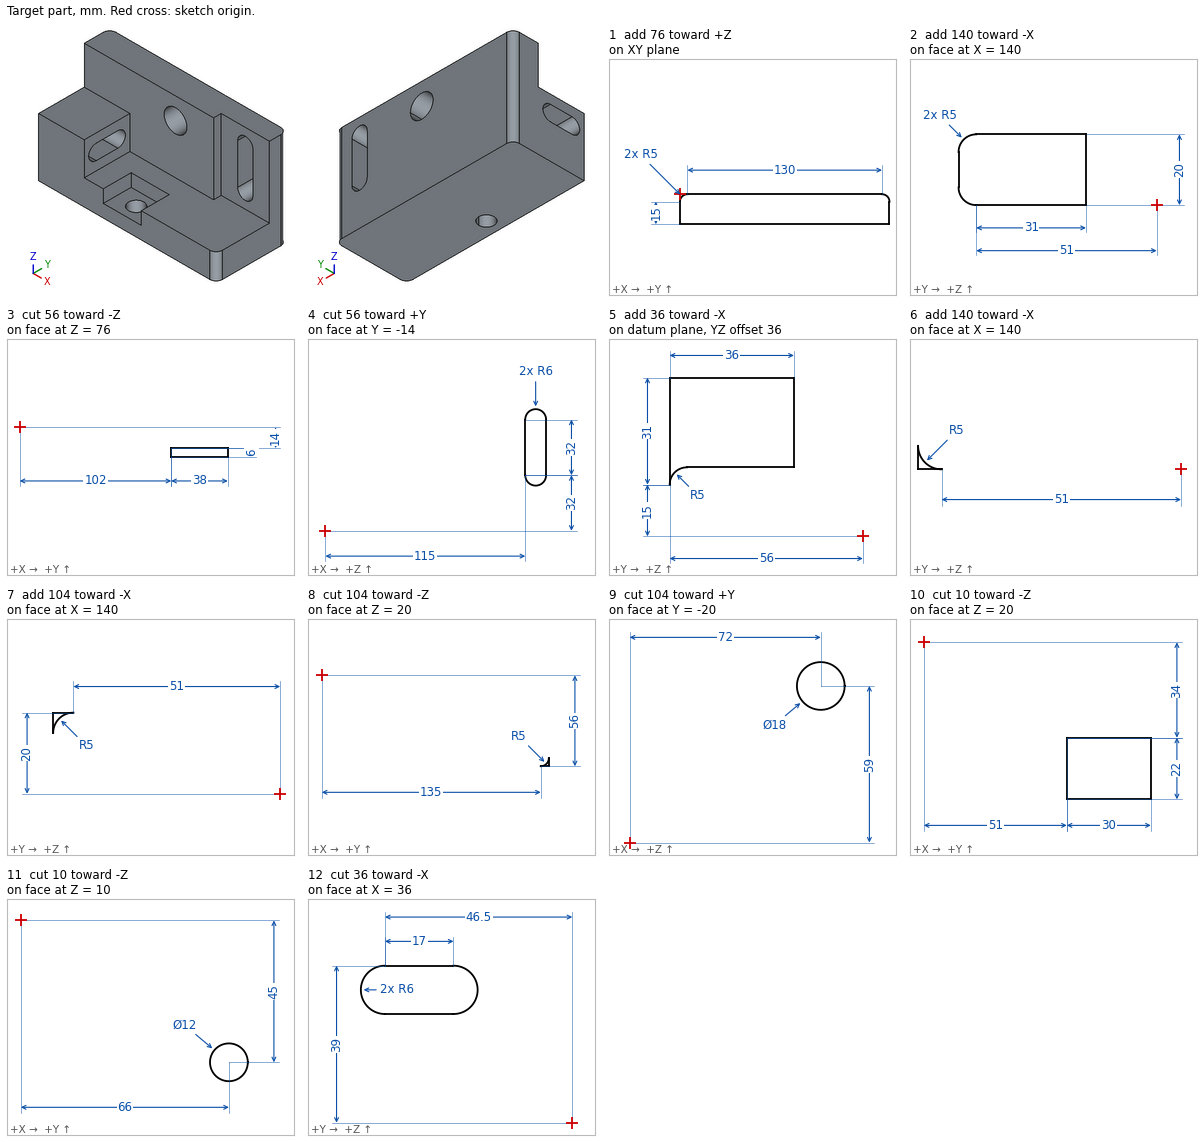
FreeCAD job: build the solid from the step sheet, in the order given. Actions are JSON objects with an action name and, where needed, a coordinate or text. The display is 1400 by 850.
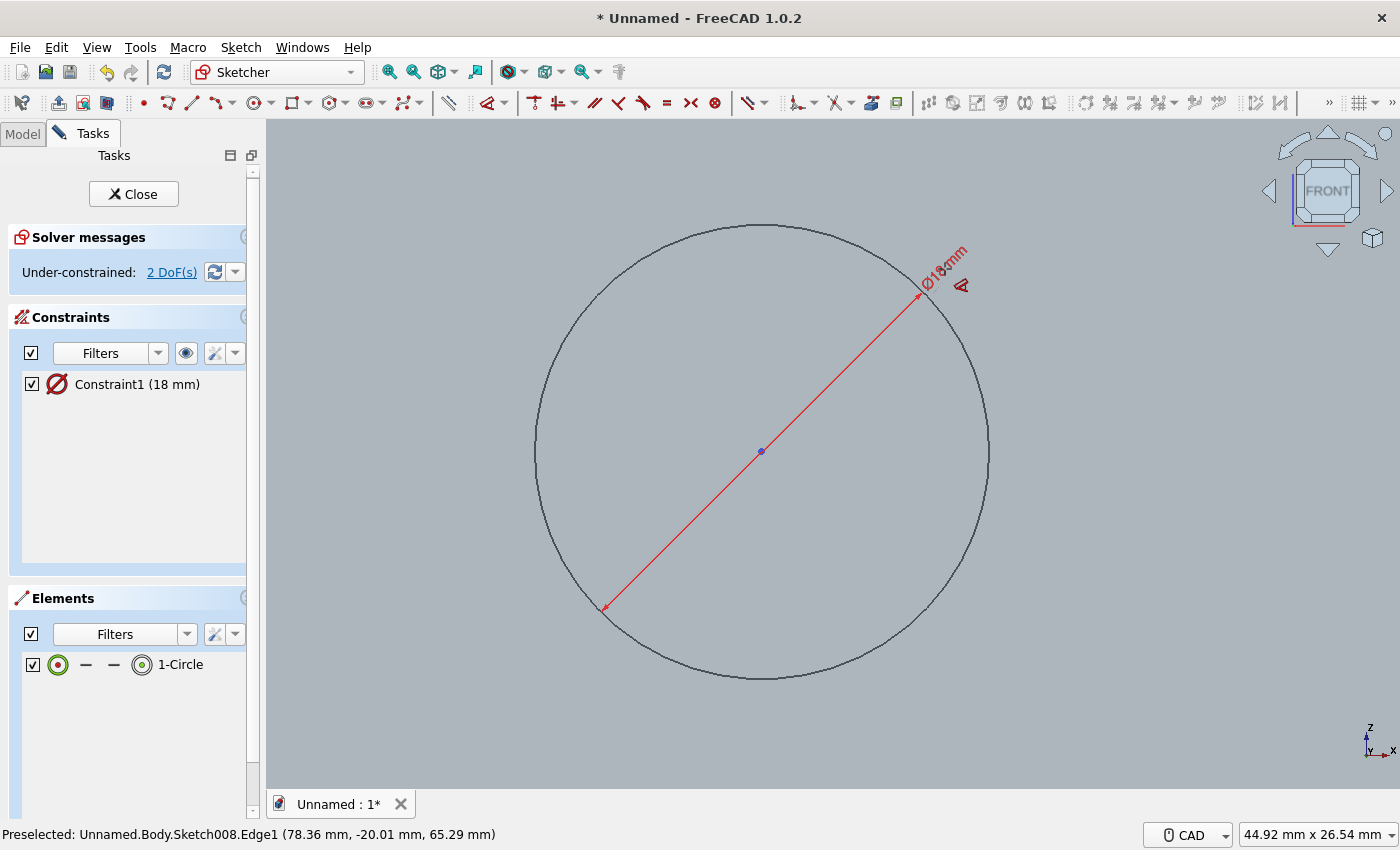
{"action": "left_click", "coordinate": [762, 452]}
{"action": "left_click", "coordinate": [420, 418]}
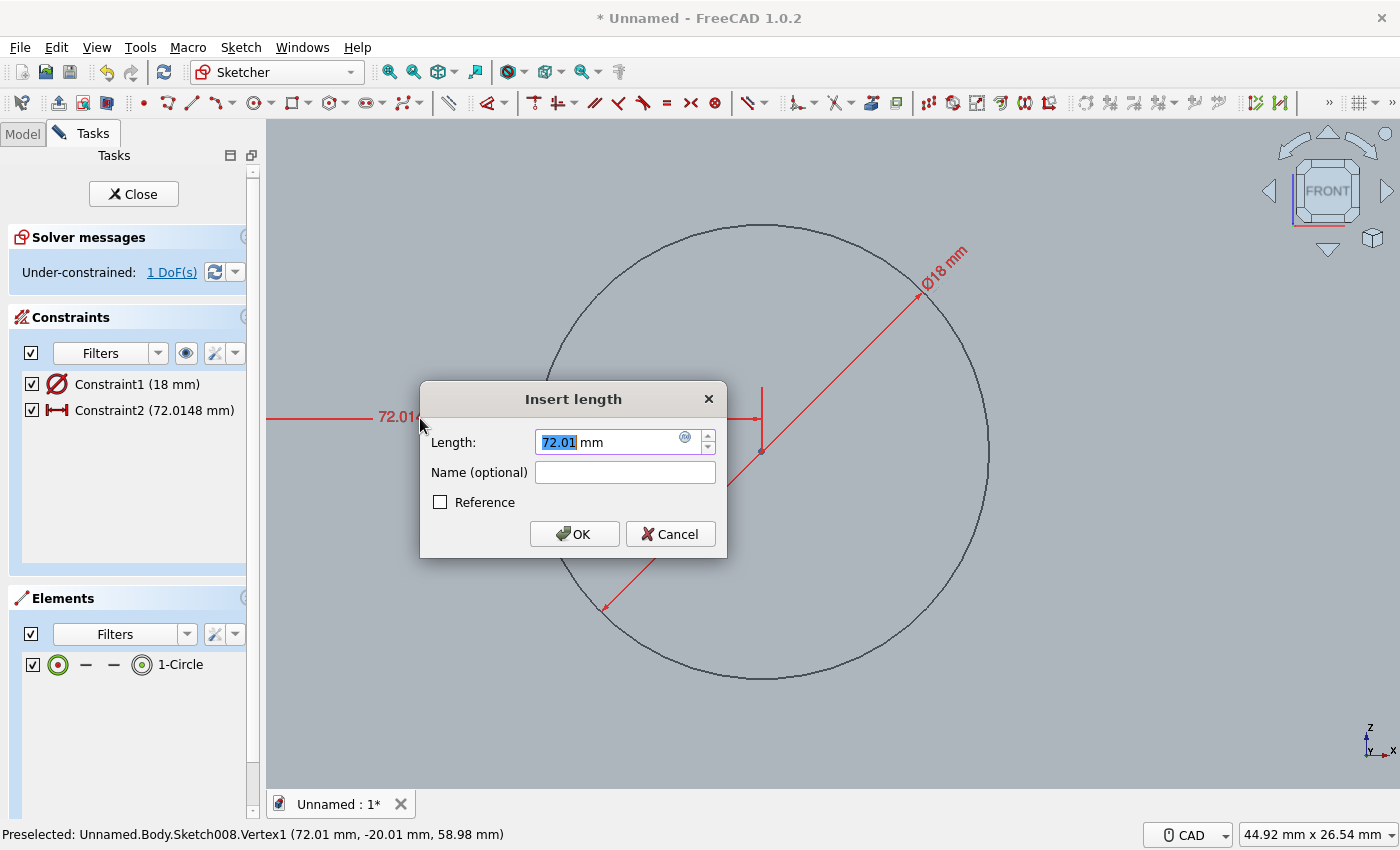
{"action": "type", "text": "72"}
{"action": "key", "text": "Return"}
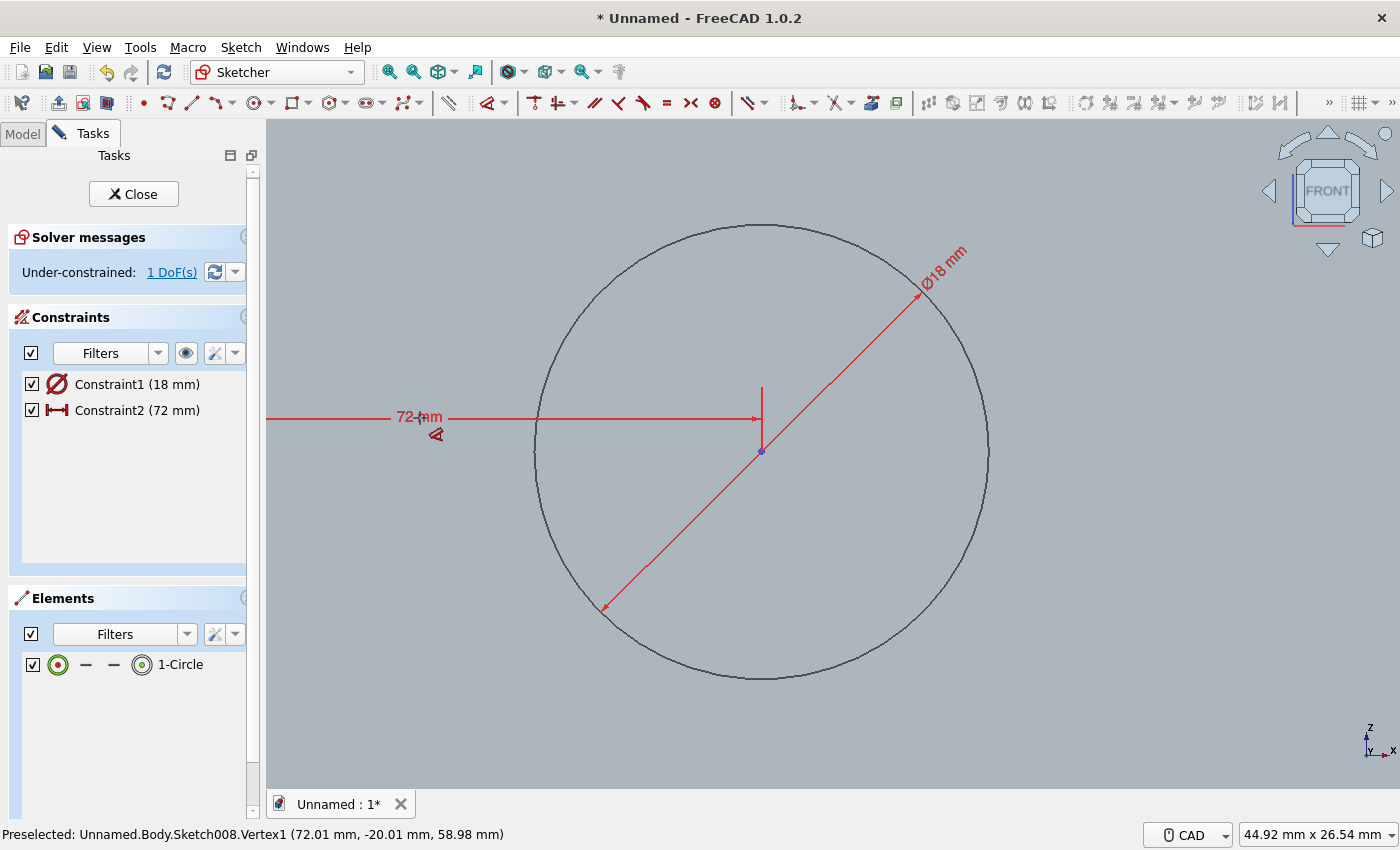
{"action": "left_click", "coordinate": [762, 452]}
{"action": "left_click", "coordinate": [796, 606]}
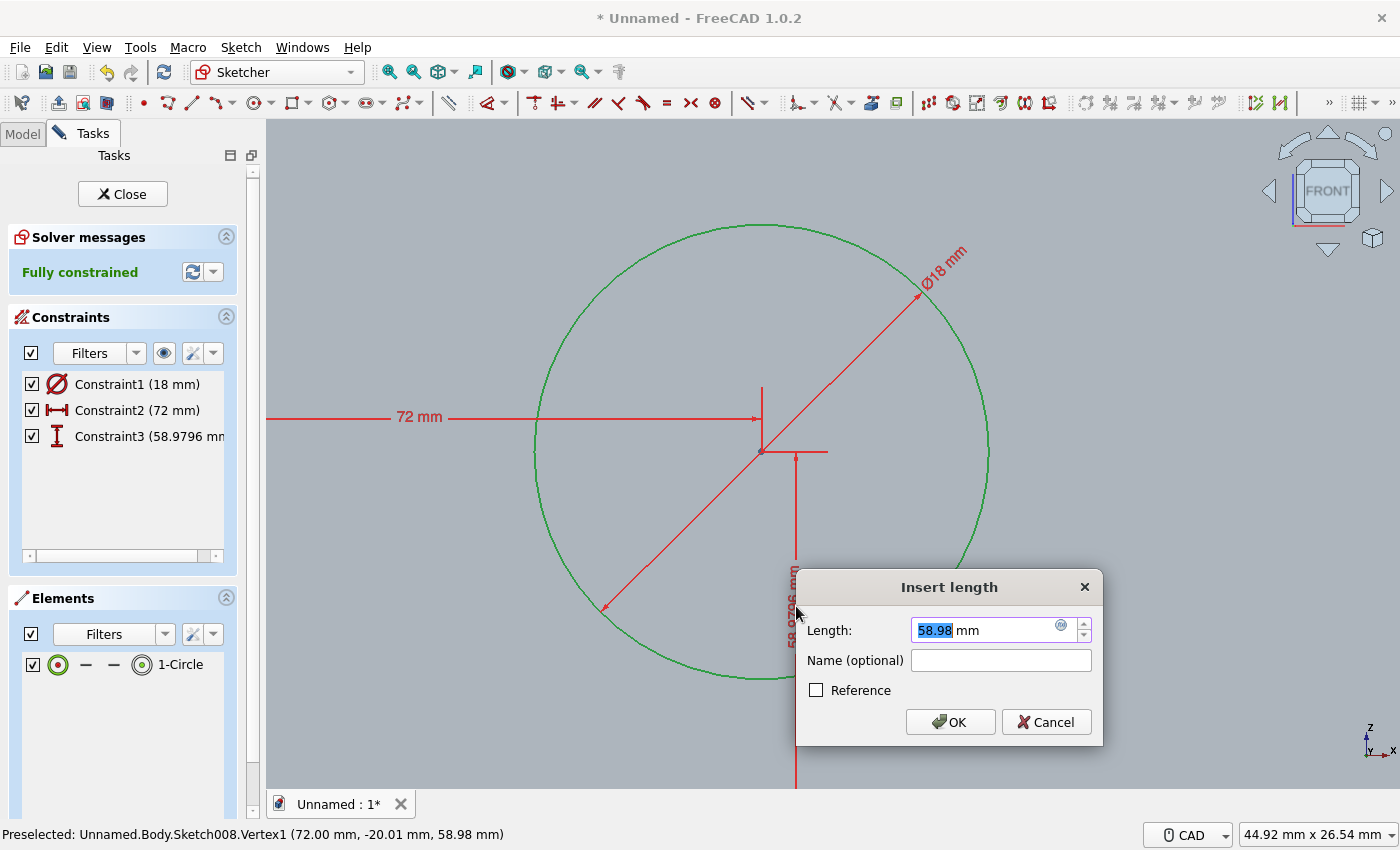
{"action": "type", "text": "59"}
{"action": "key", "text": "Return"}
{"action": "key", "text": "Escape"}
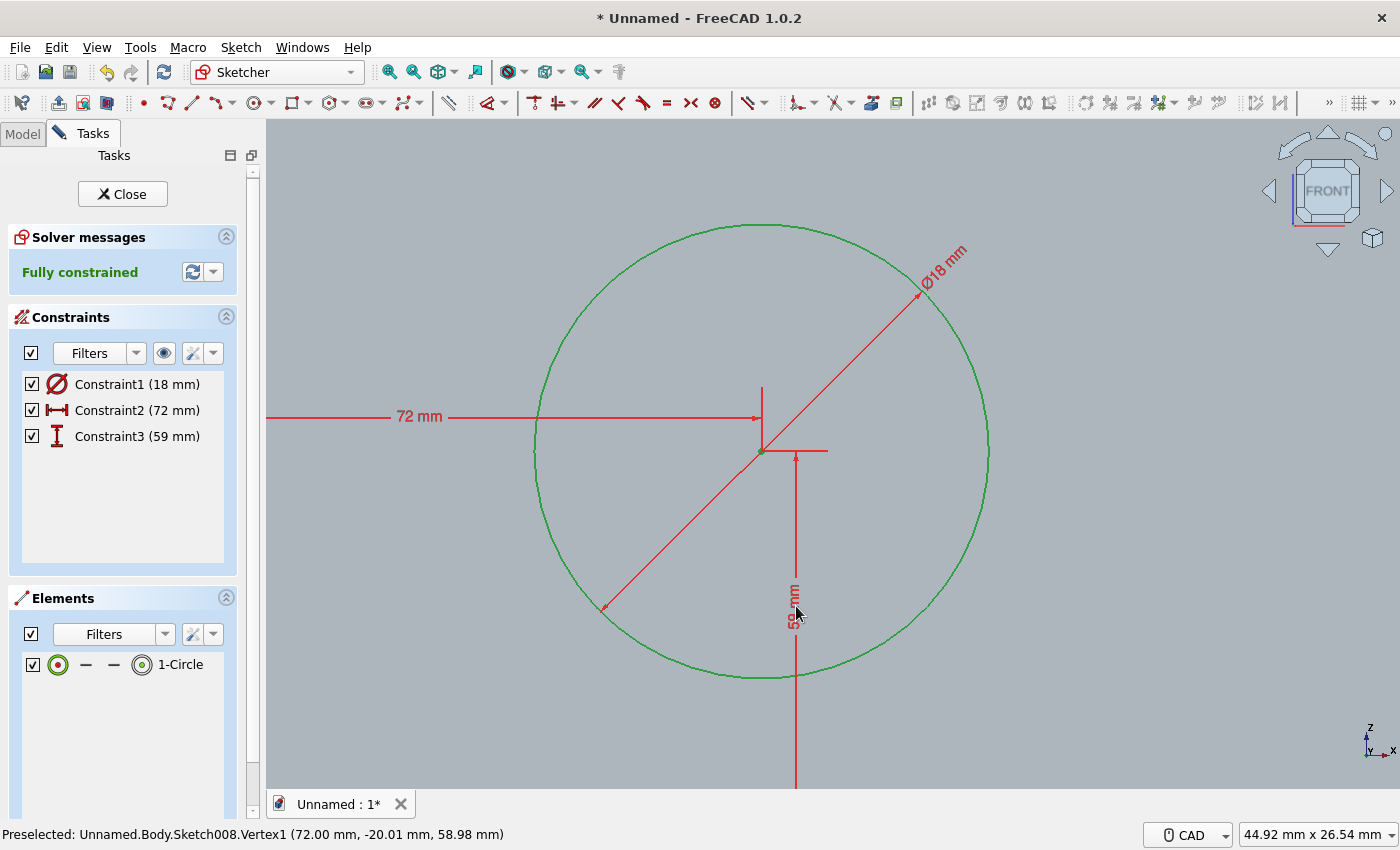
{"action": "left_click", "coordinate": [123, 194]}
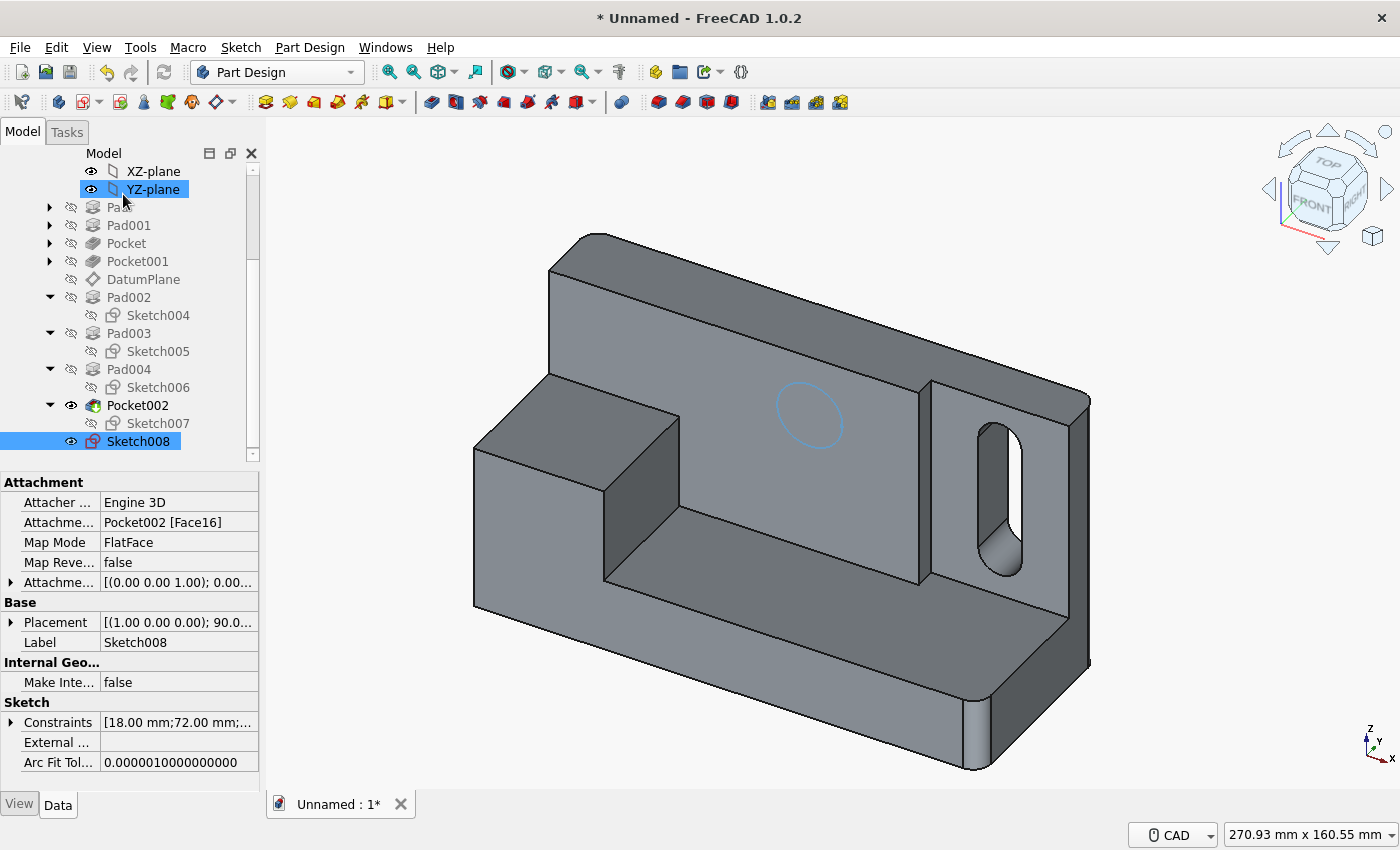
{"action": "left_click", "coordinate": [432, 102]}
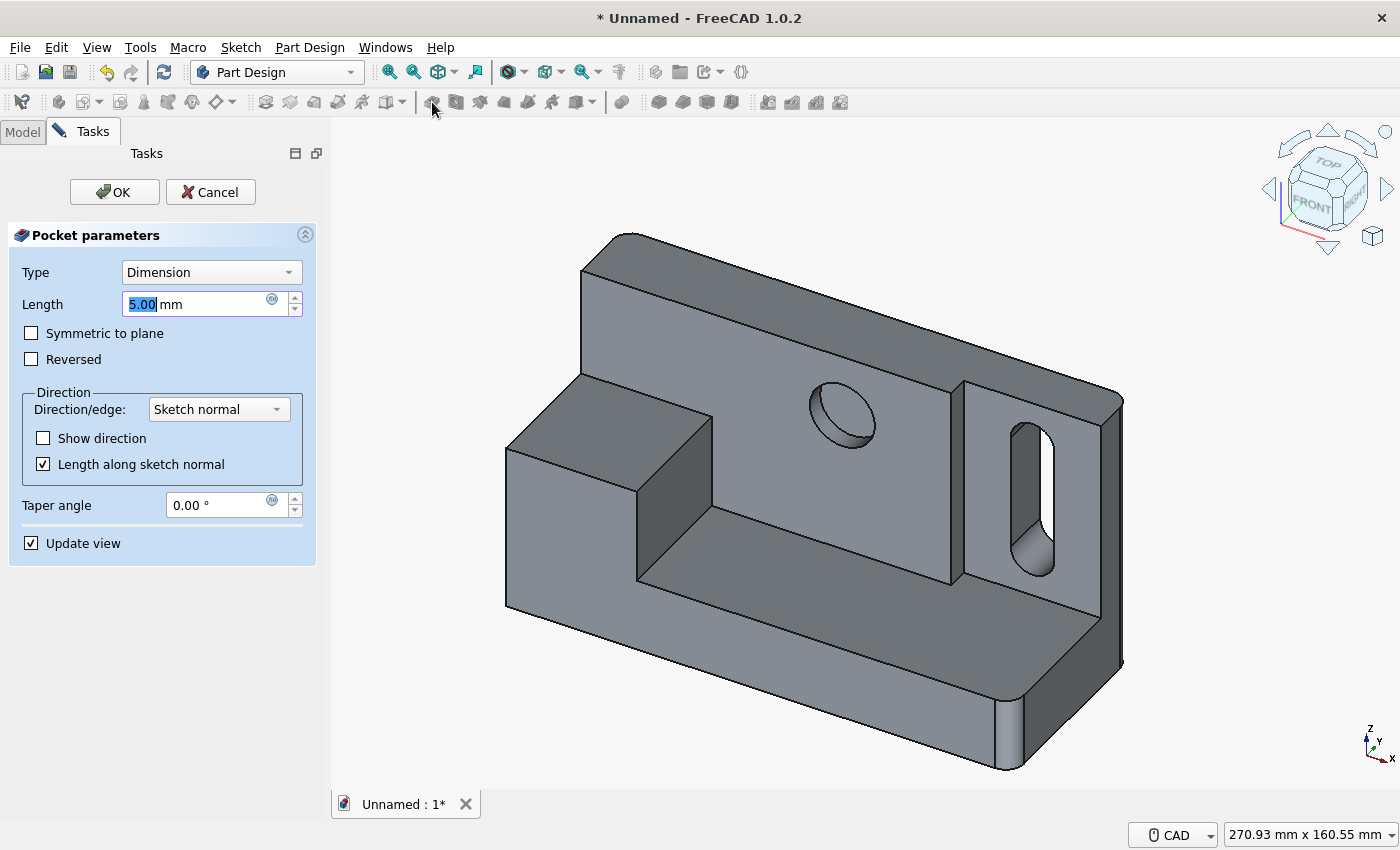
{"action": "type", "text": "104"}
{"action": "key", "text": "Tab"}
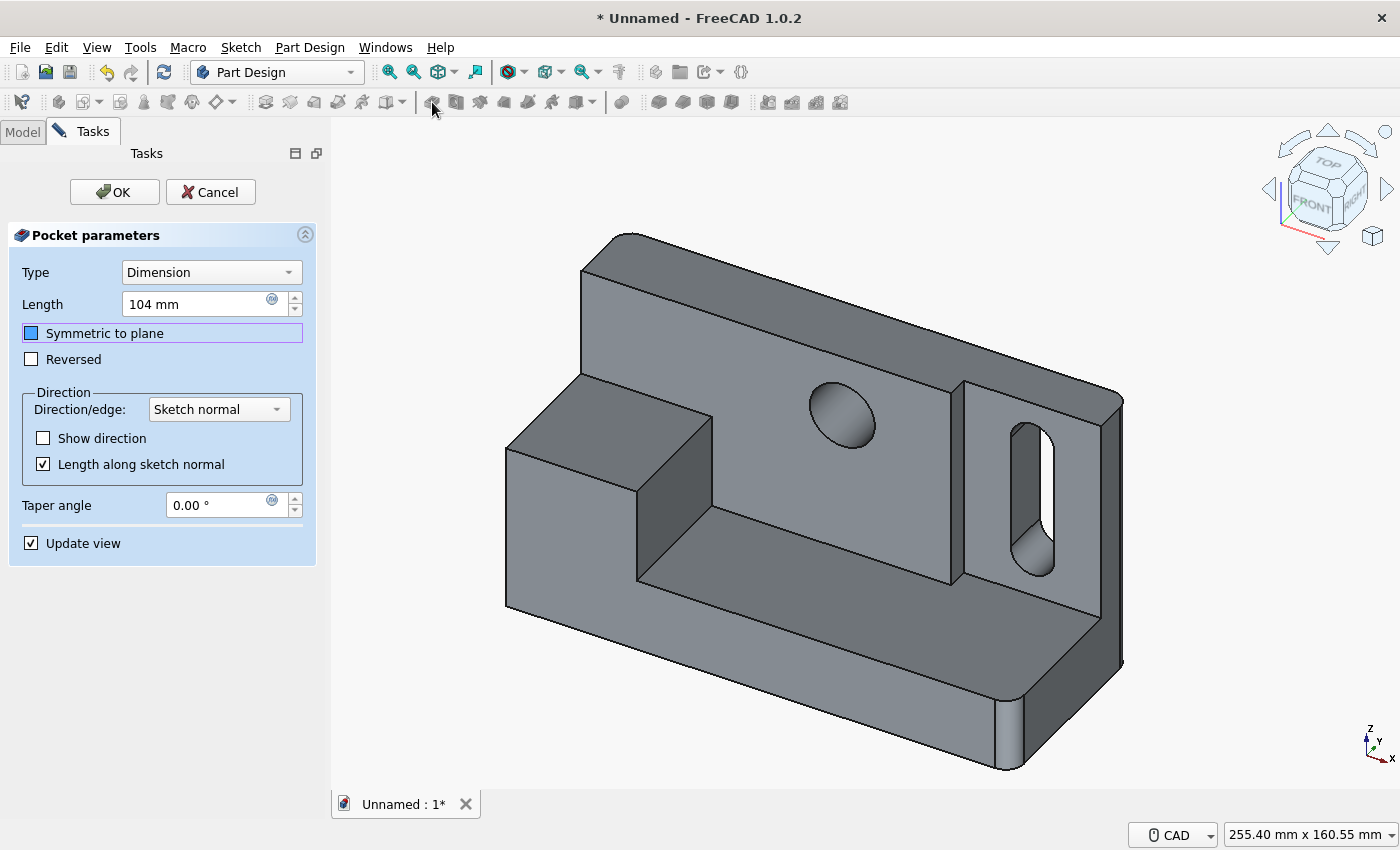
{"action": "left_click", "coordinate": [115, 192]}